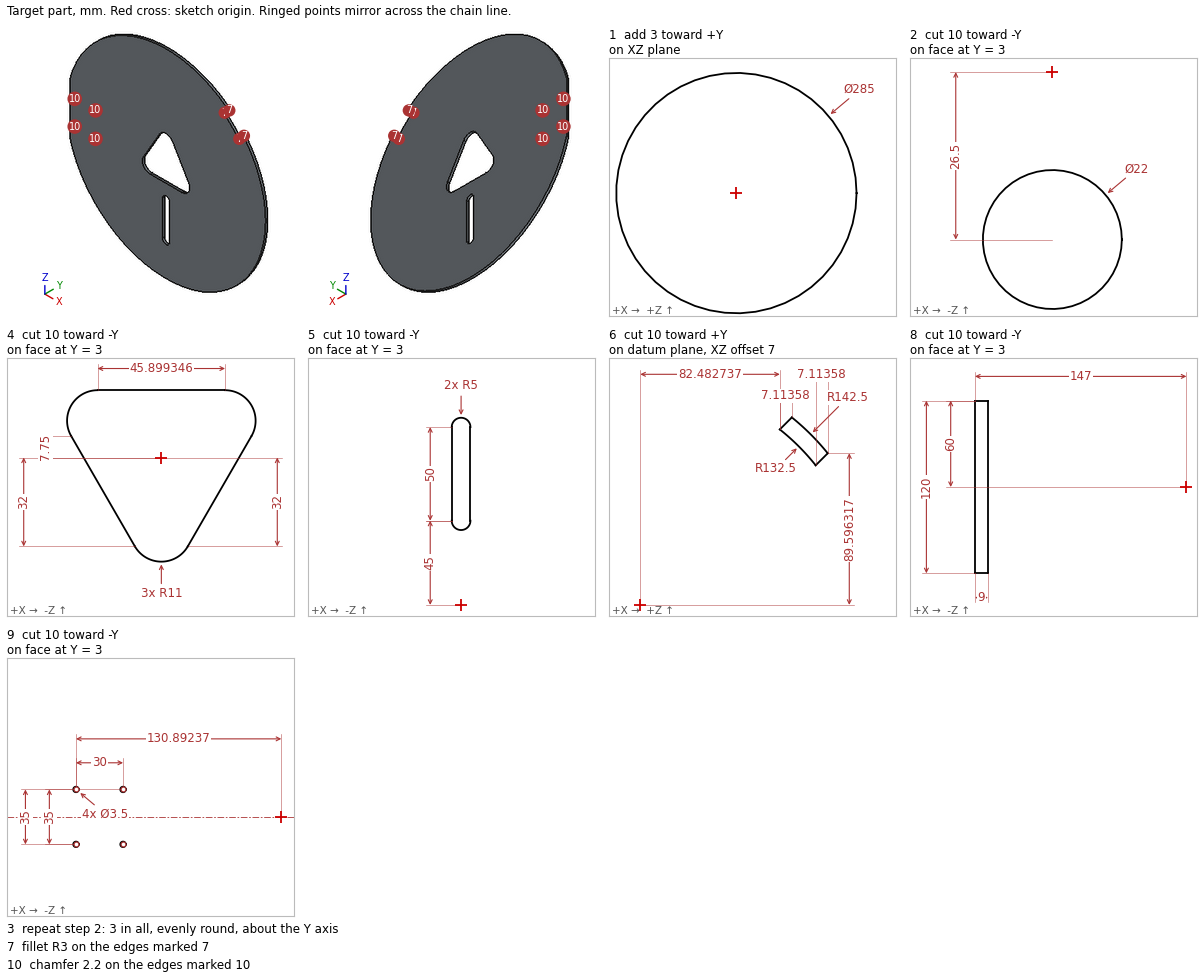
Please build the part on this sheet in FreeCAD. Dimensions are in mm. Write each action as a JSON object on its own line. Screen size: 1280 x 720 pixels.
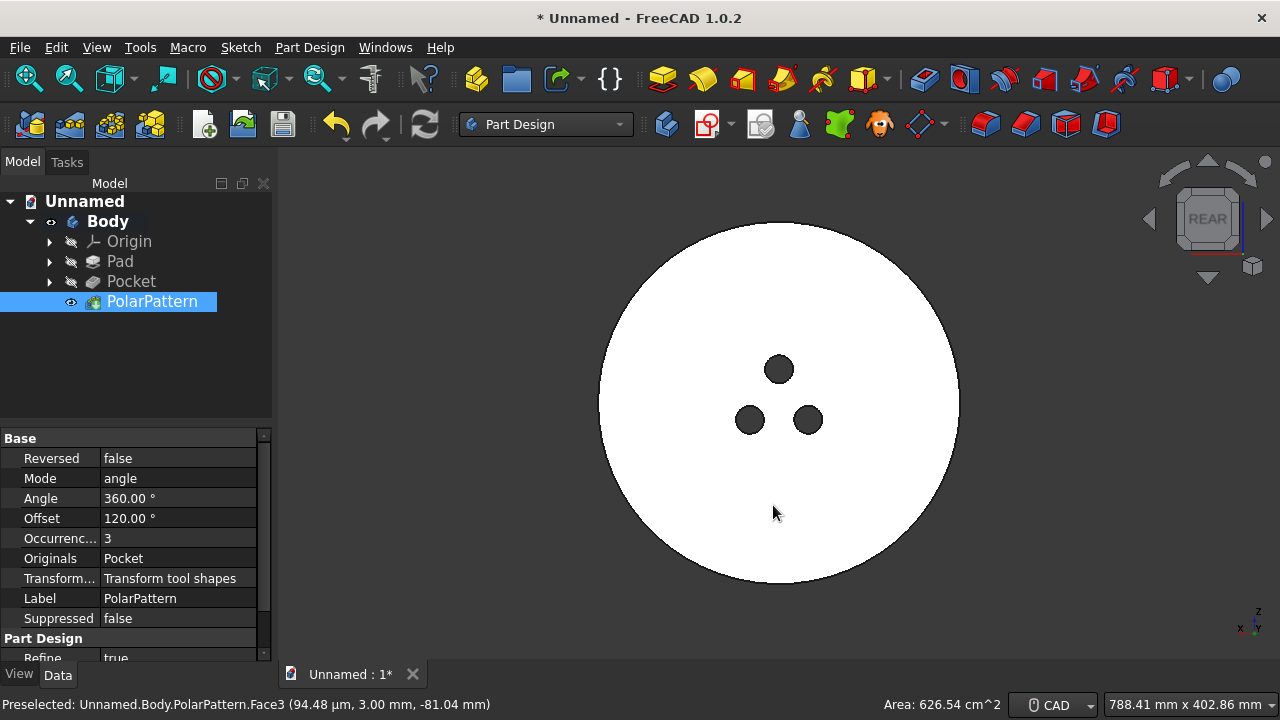
{"action": "left_click", "coordinate": [708, 124]}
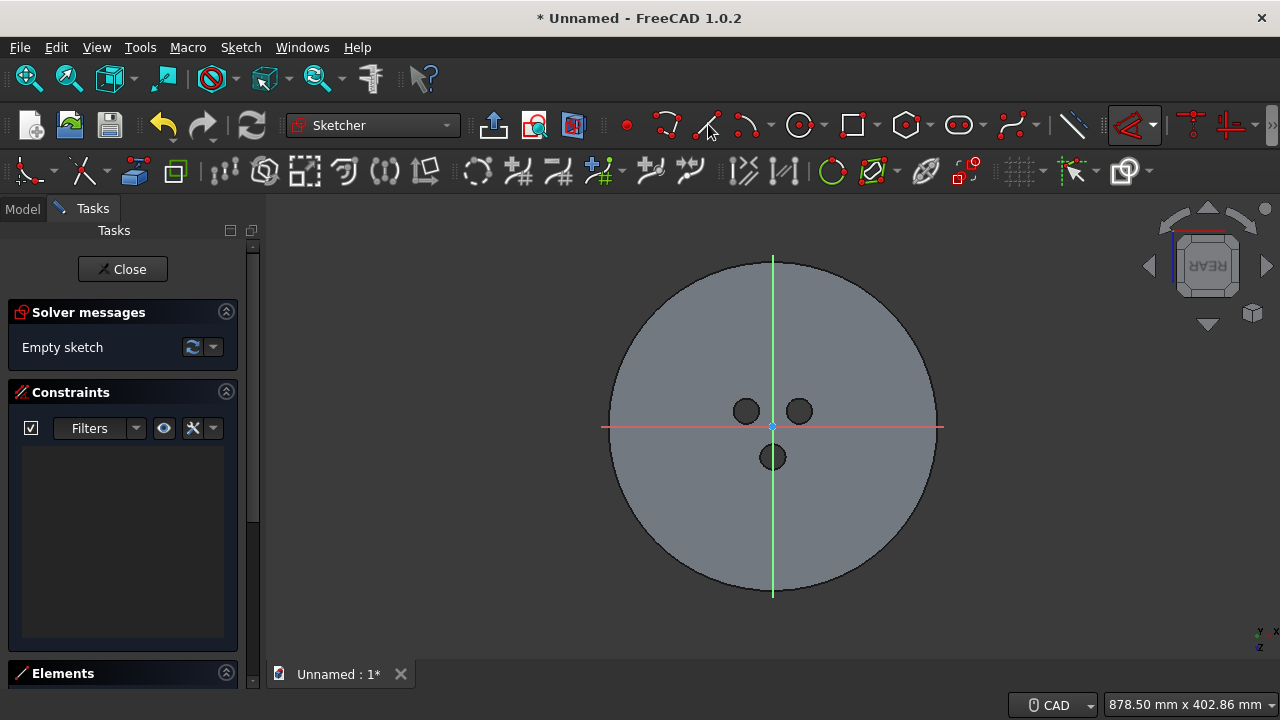
{"action": "scroll", "coordinate": [795, 437], "scroll_direction": "up", "scroll_amount": 7}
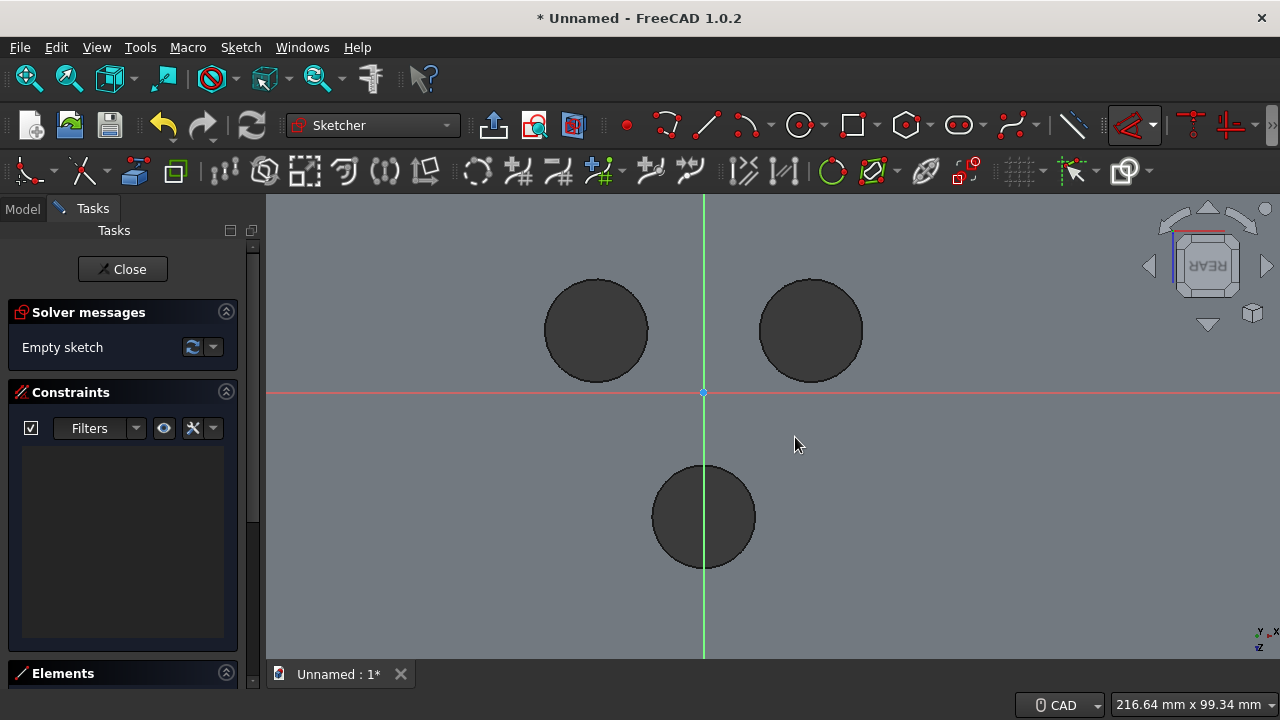
{"action": "key", "text": "g l"}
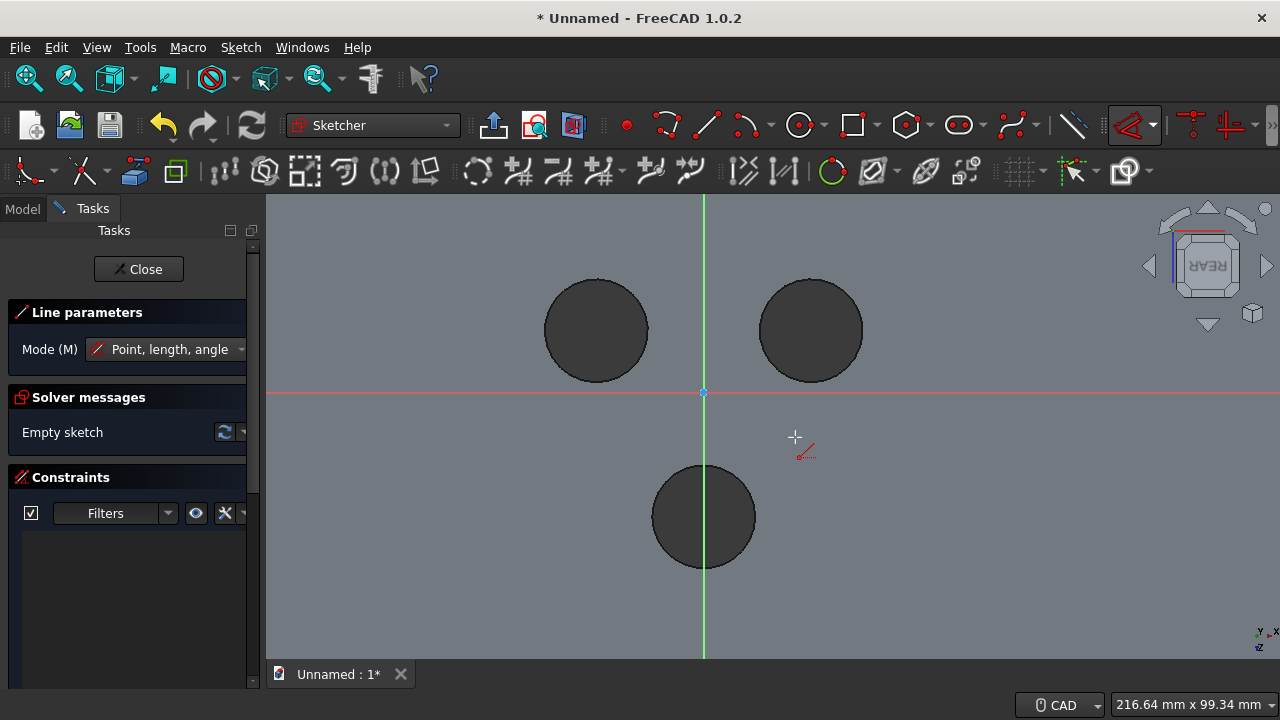
{"action": "left_click", "coordinate": [552, 357]}
{"action": "left_click", "coordinate": [659, 543]}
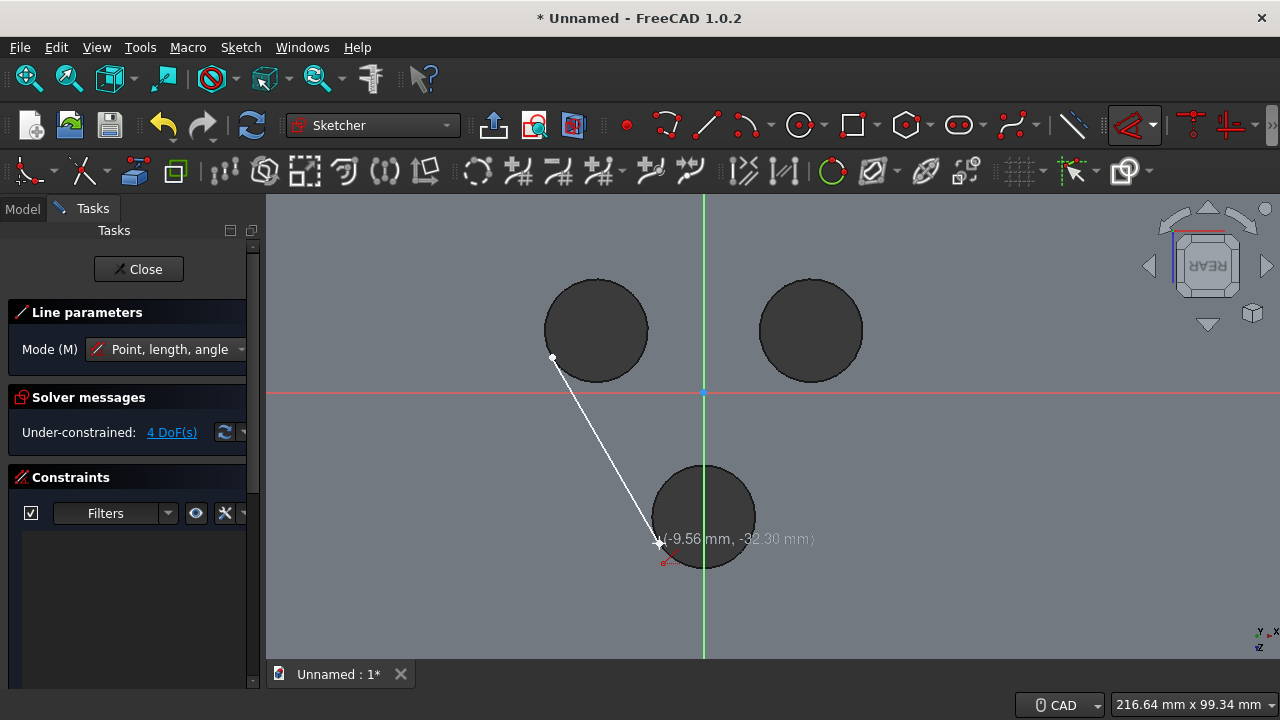
{"action": "left_click", "coordinate": [748, 543]}
{"action": "left_click", "coordinate": [856, 357]}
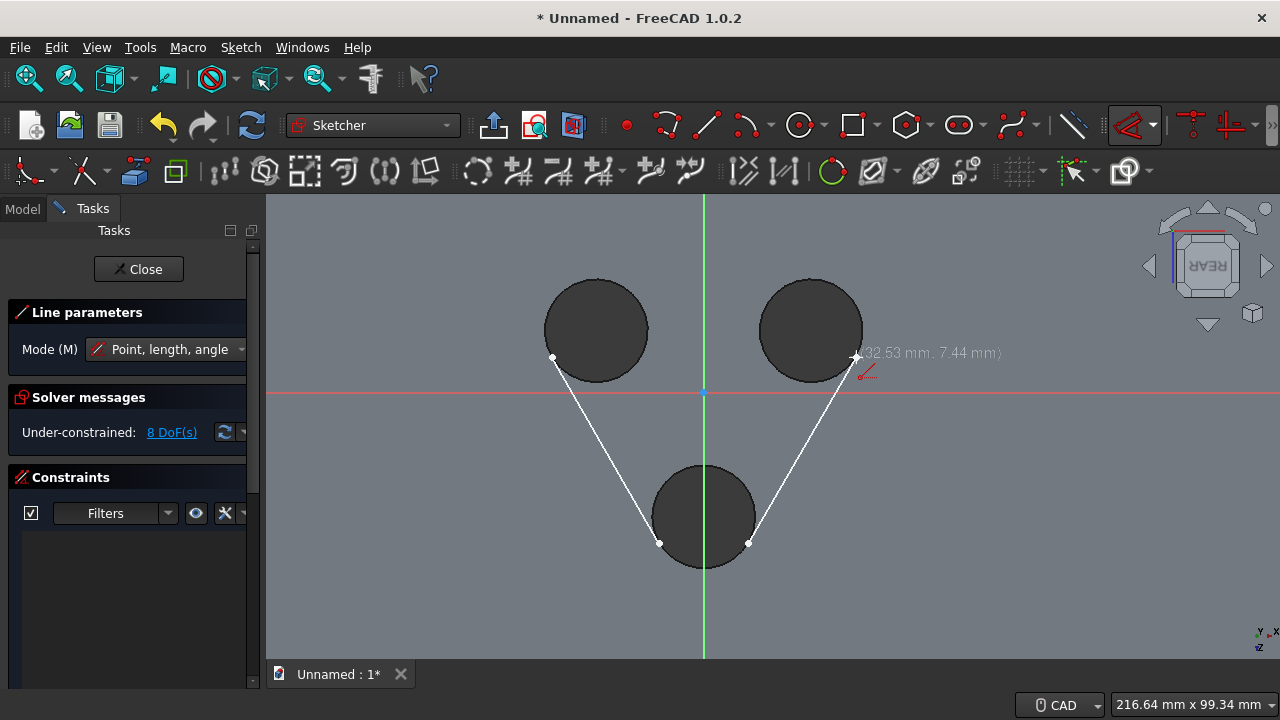
{"action": "left_click", "coordinate": [811, 279]}
{"action": "left_click", "coordinate": [596, 279]}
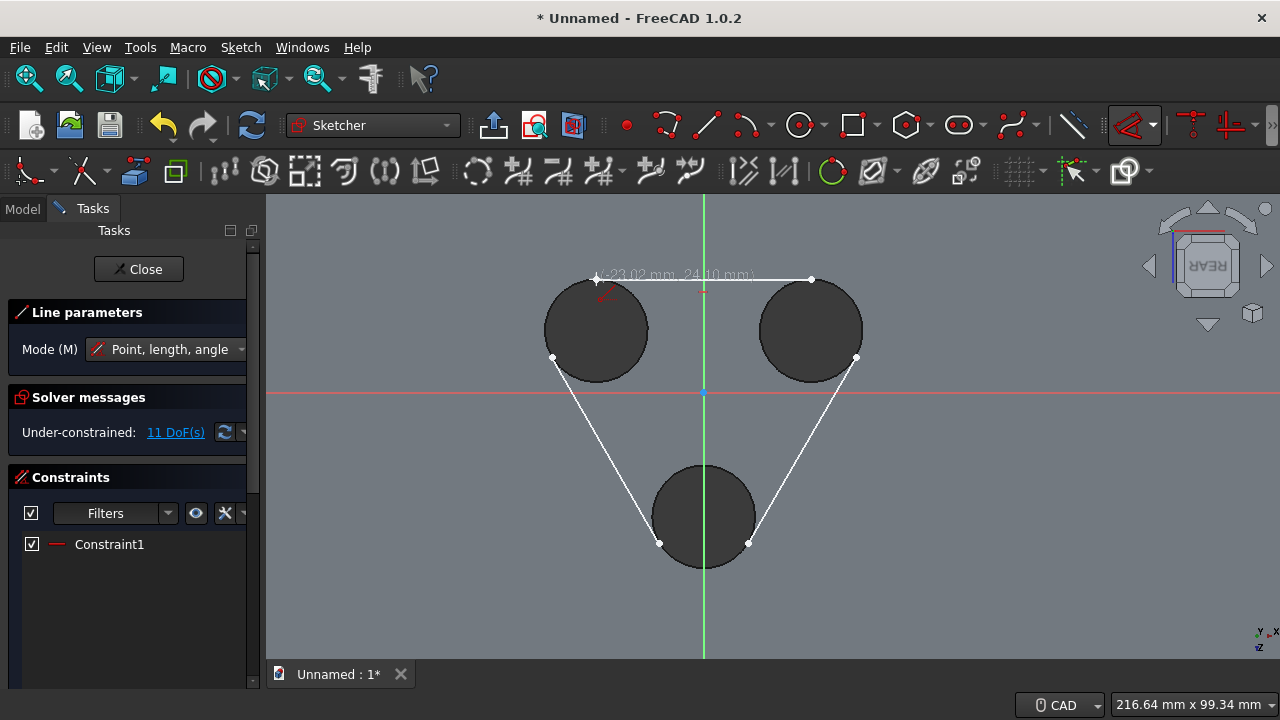
{"action": "left_click", "coordinate": [774, 126]}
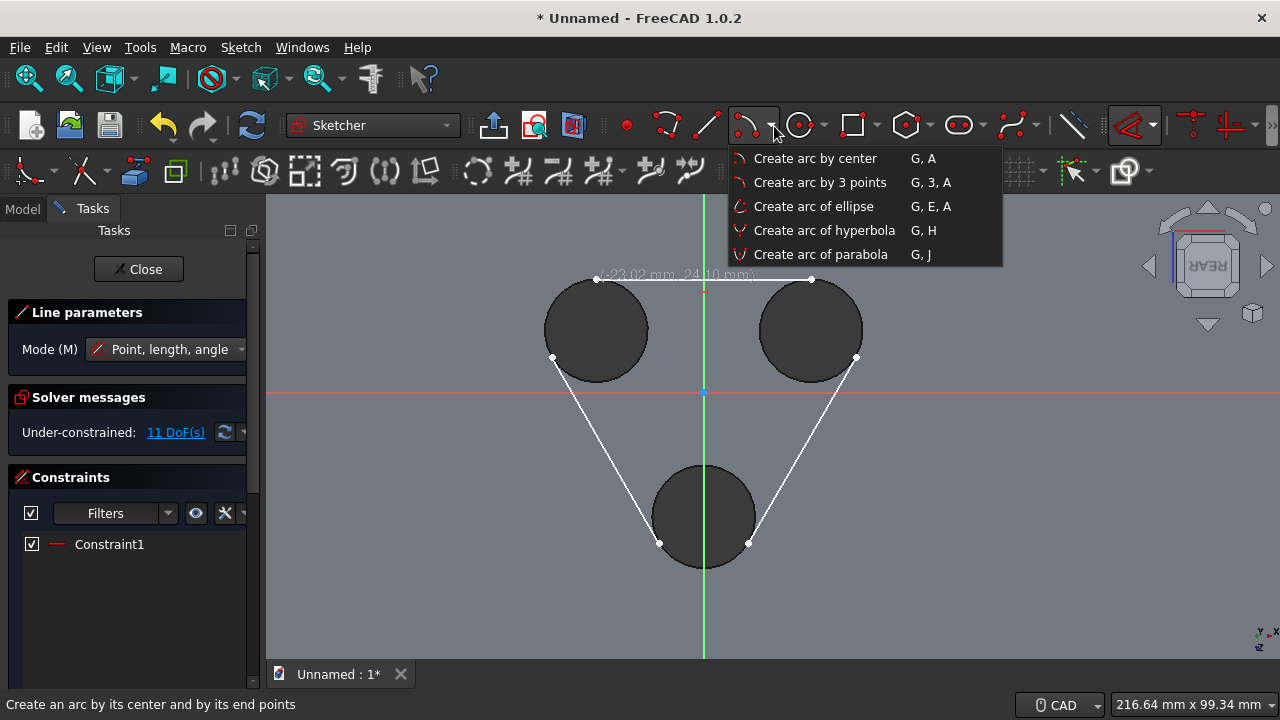
{"action": "left_click", "coordinate": [866, 182]}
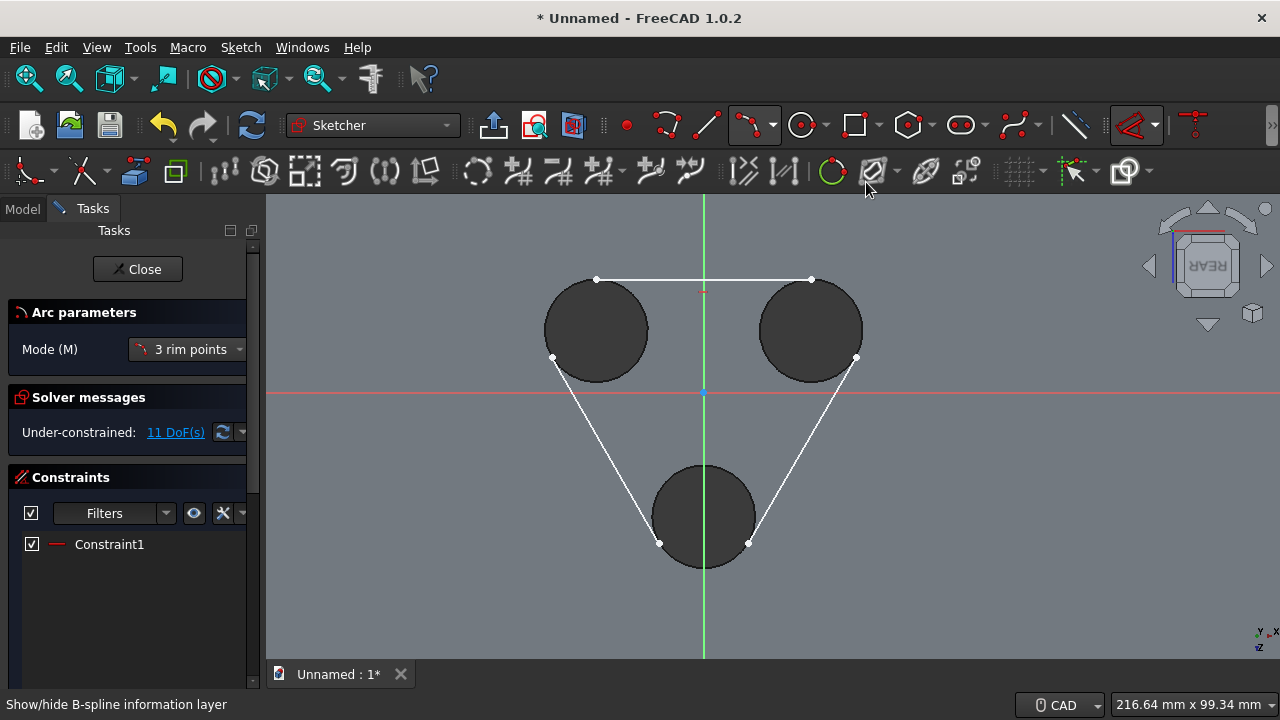
{"action": "left_click", "coordinate": [659, 544]}
{"action": "left_click", "coordinate": [748, 544]}
{"action": "left_click", "coordinate": [683, 564]}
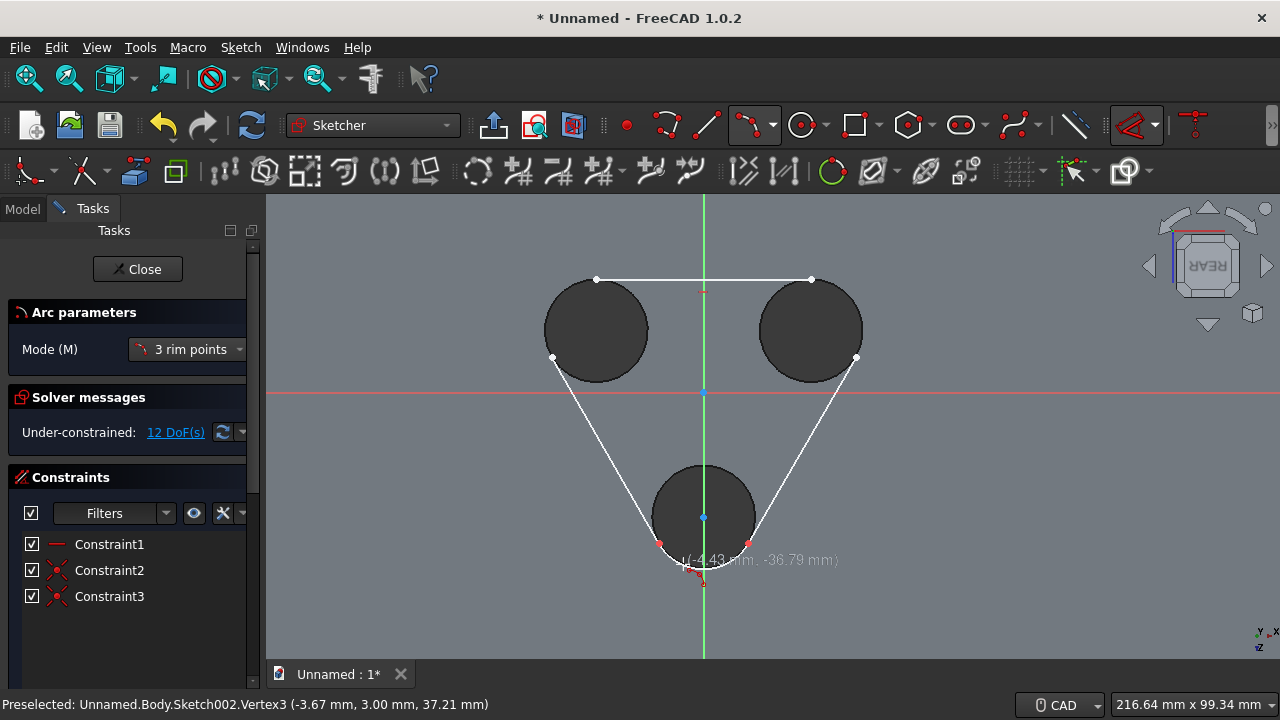
{"action": "left_click", "coordinate": [856, 358]}
{"action": "left_click", "coordinate": [811, 280]}
{"action": "left_click", "coordinate": [856, 305]}